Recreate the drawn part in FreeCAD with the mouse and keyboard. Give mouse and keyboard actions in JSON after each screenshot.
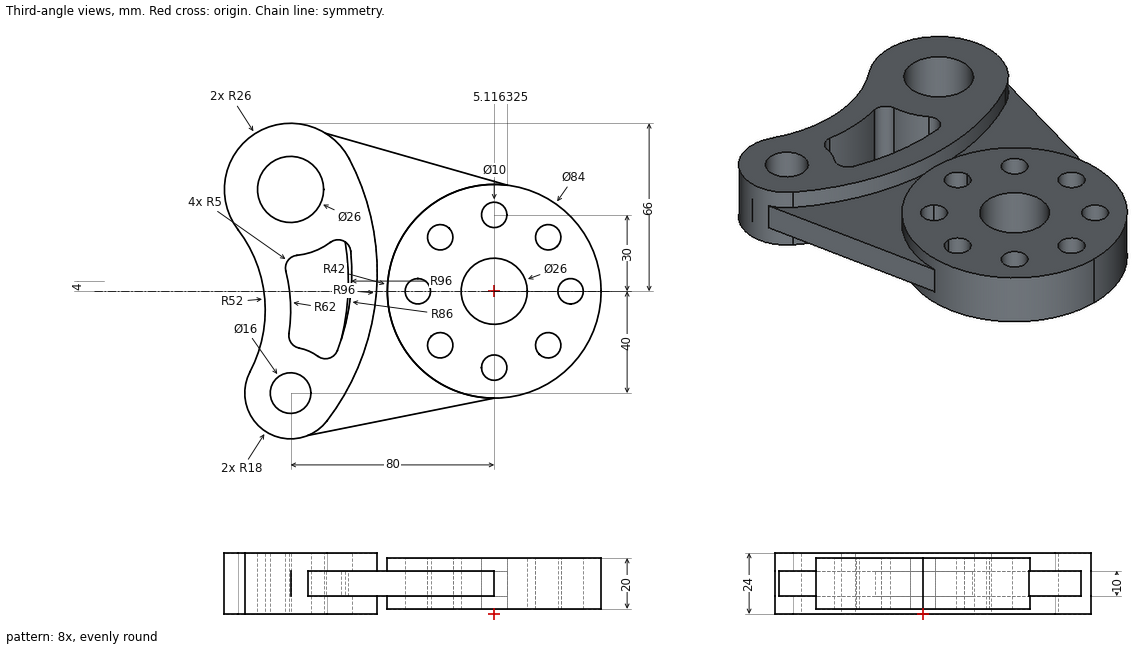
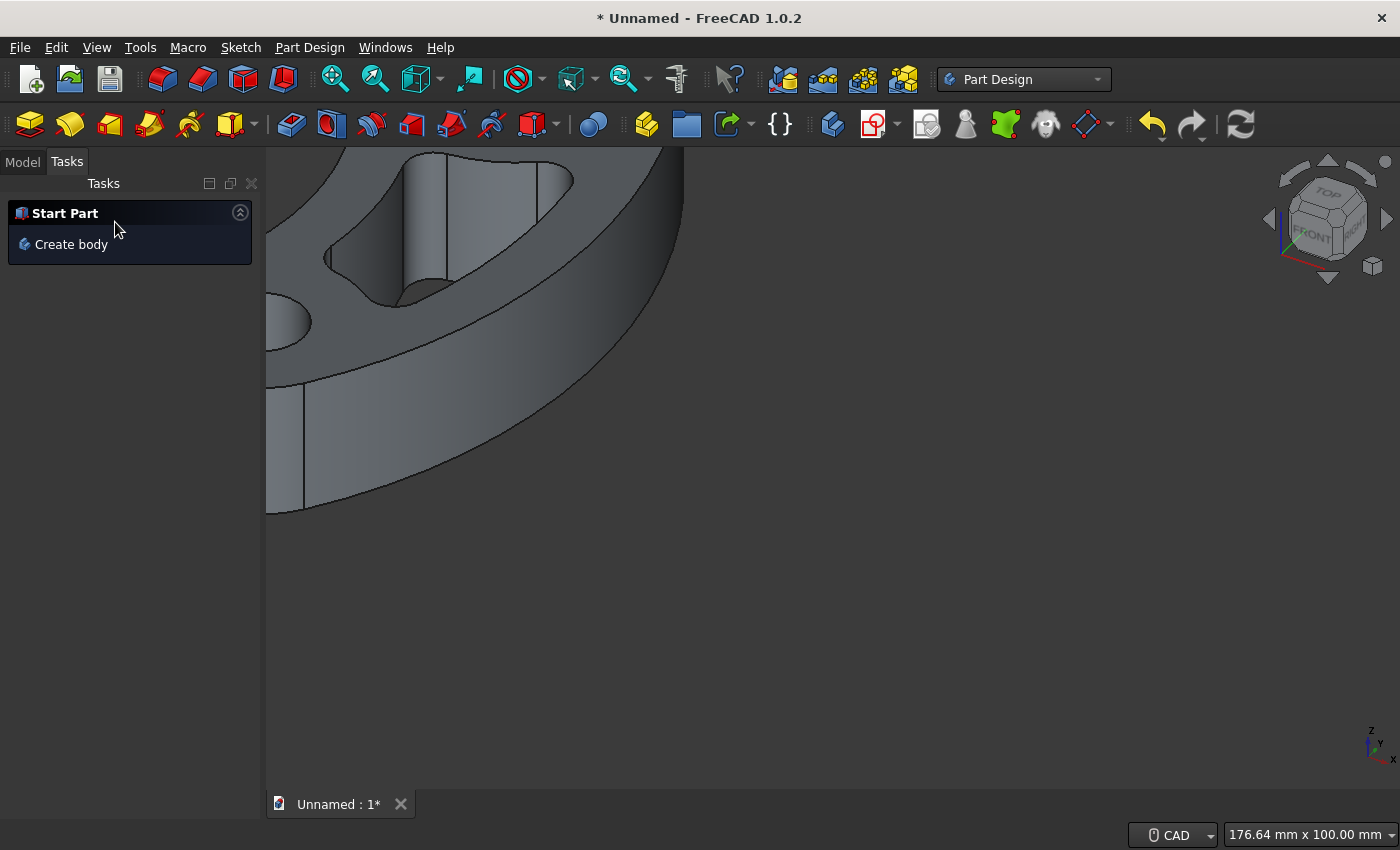
{"action": "left_click", "coordinate": [336, 80]}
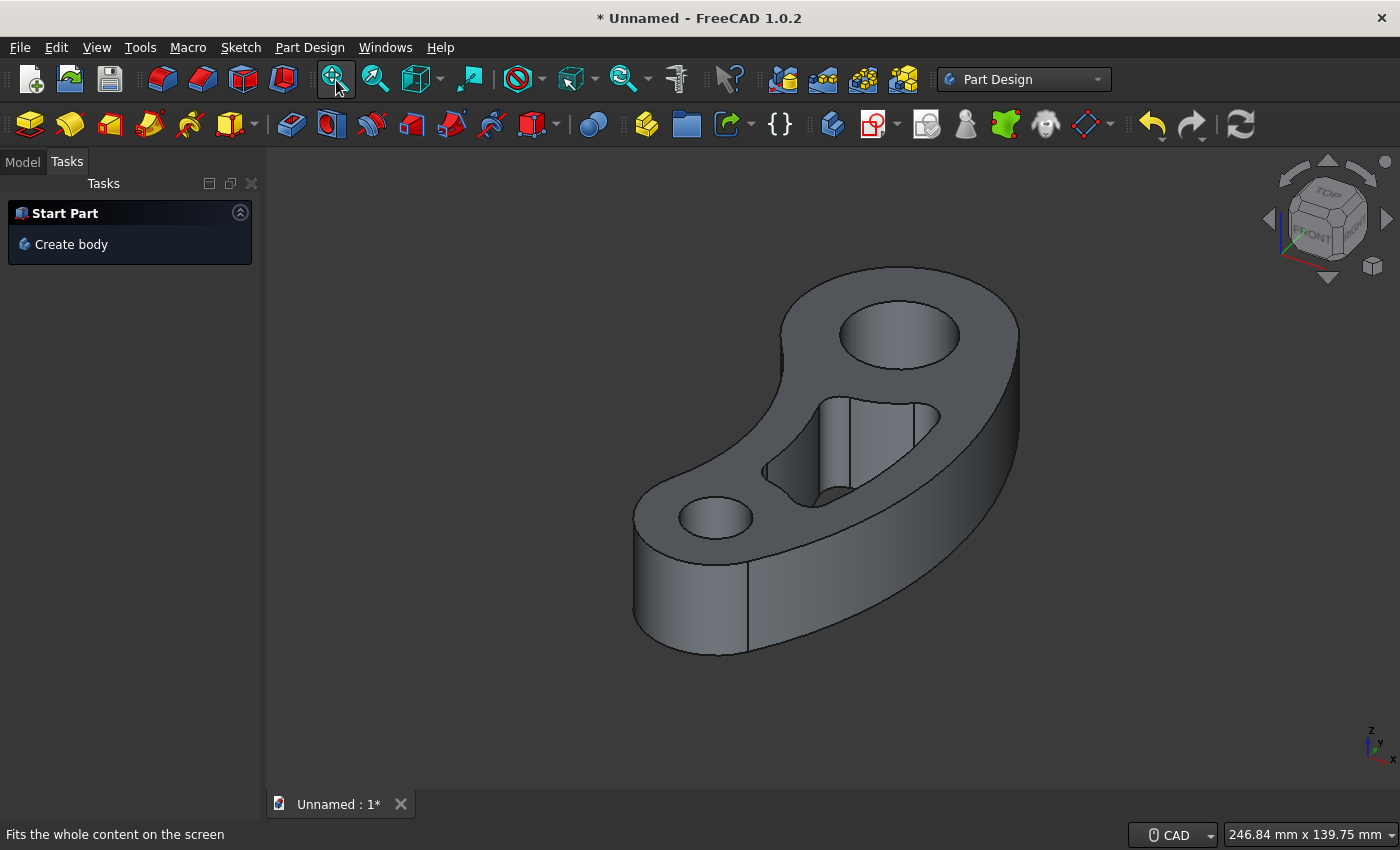
{"action": "left_click", "coordinate": [834, 124]}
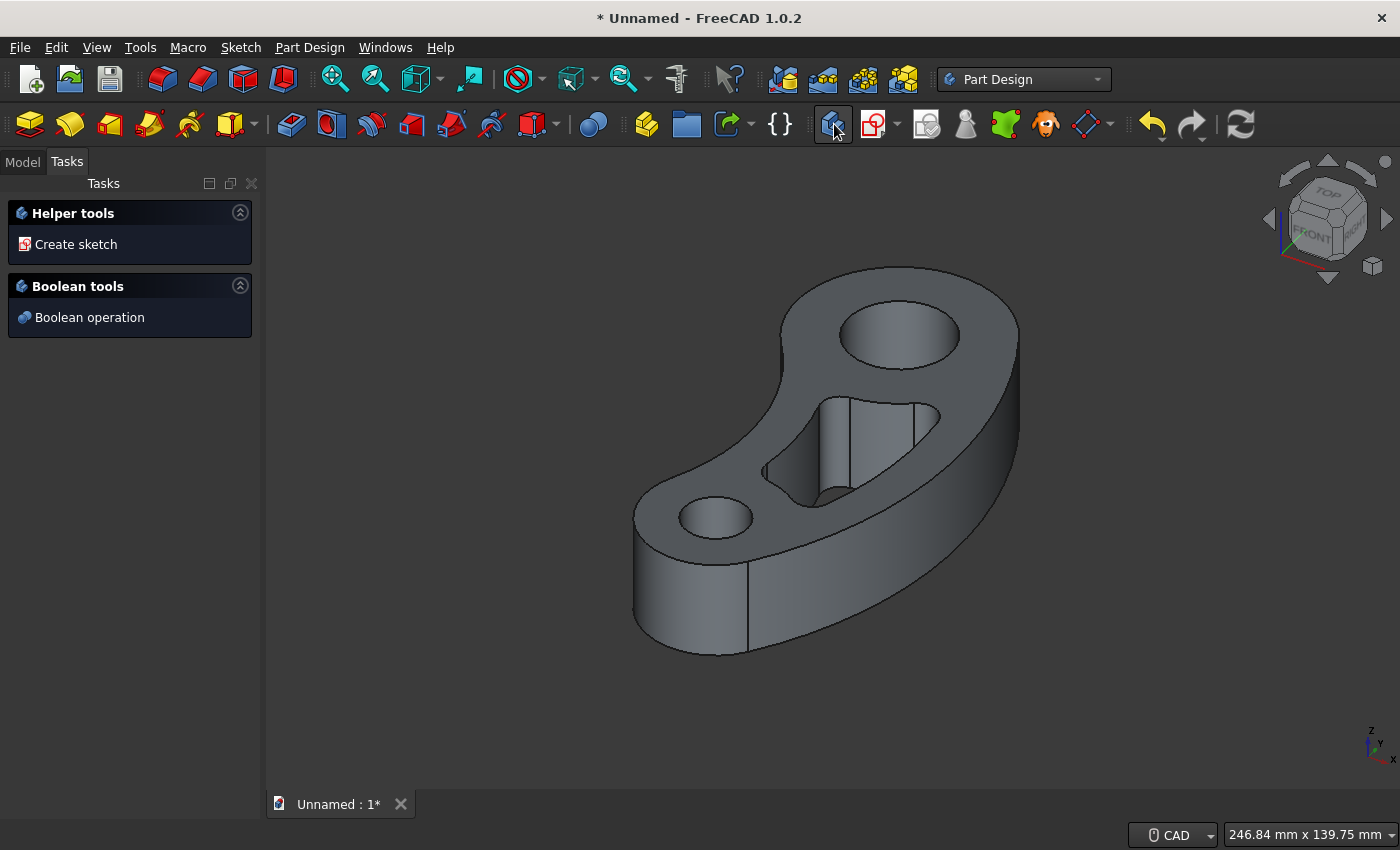
{"action": "left_click", "coordinate": [23, 161]}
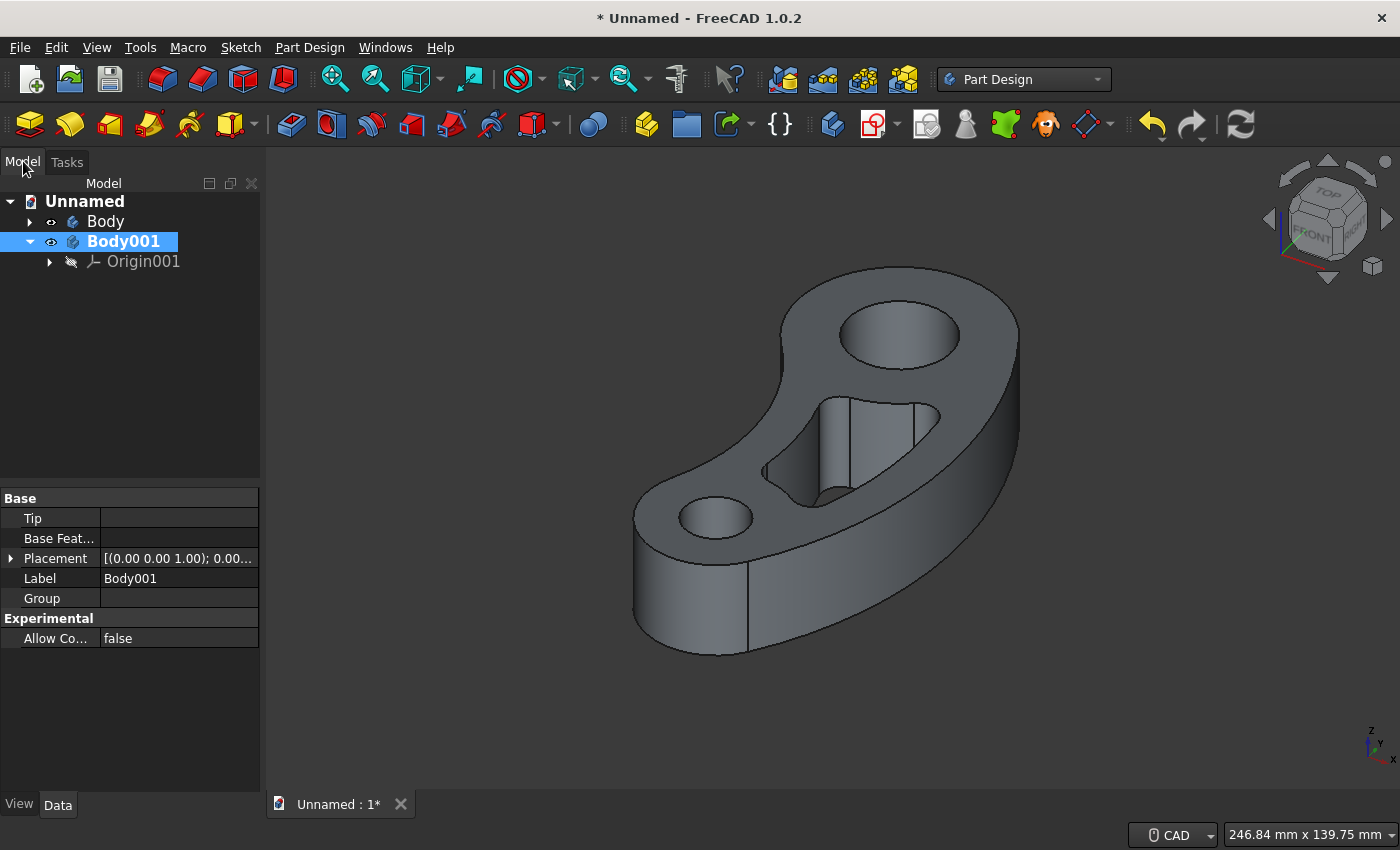
{"action": "left_click", "coordinate": [50, 262]}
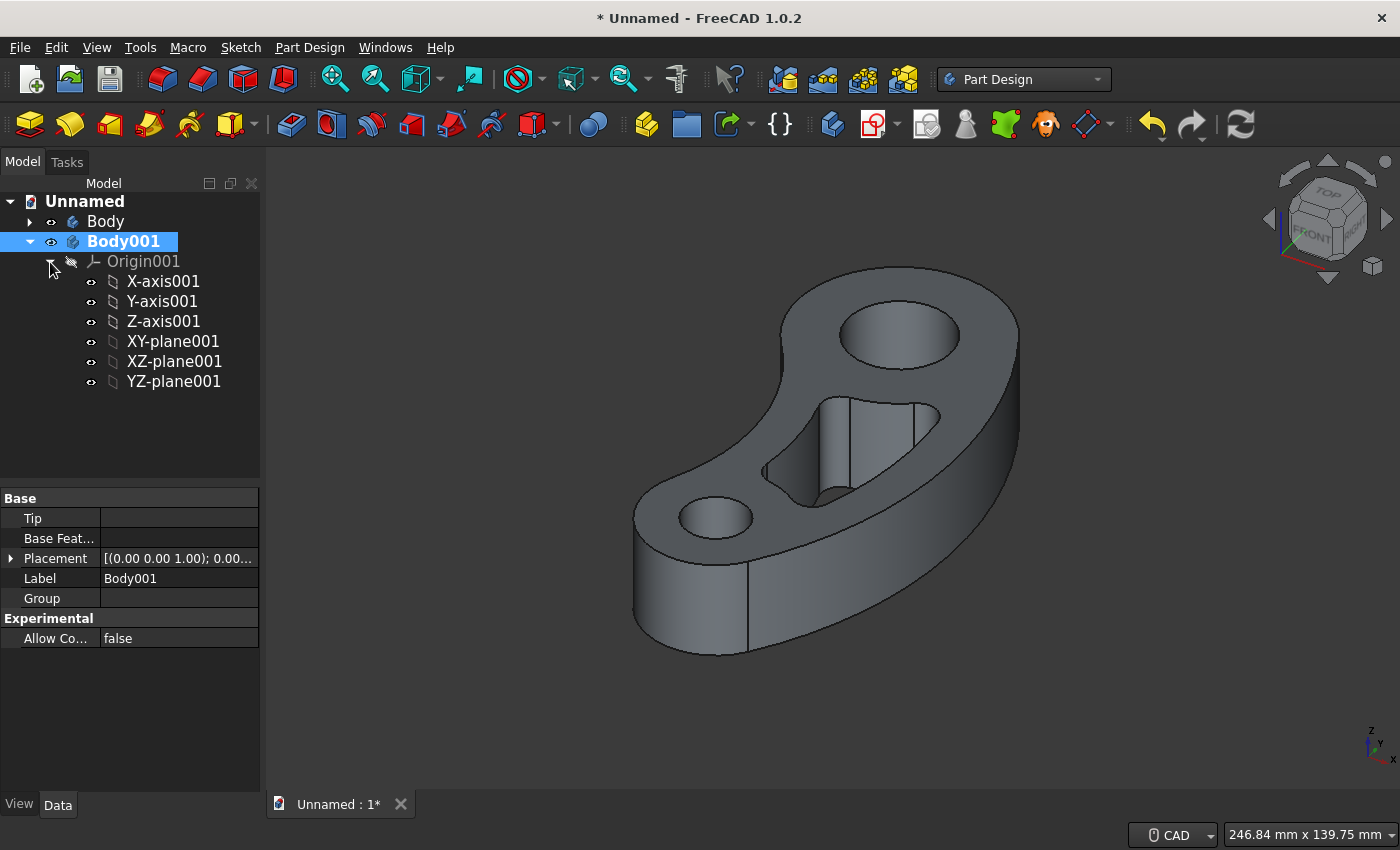
{"action": "left_click", "coordinate": [136, 342]}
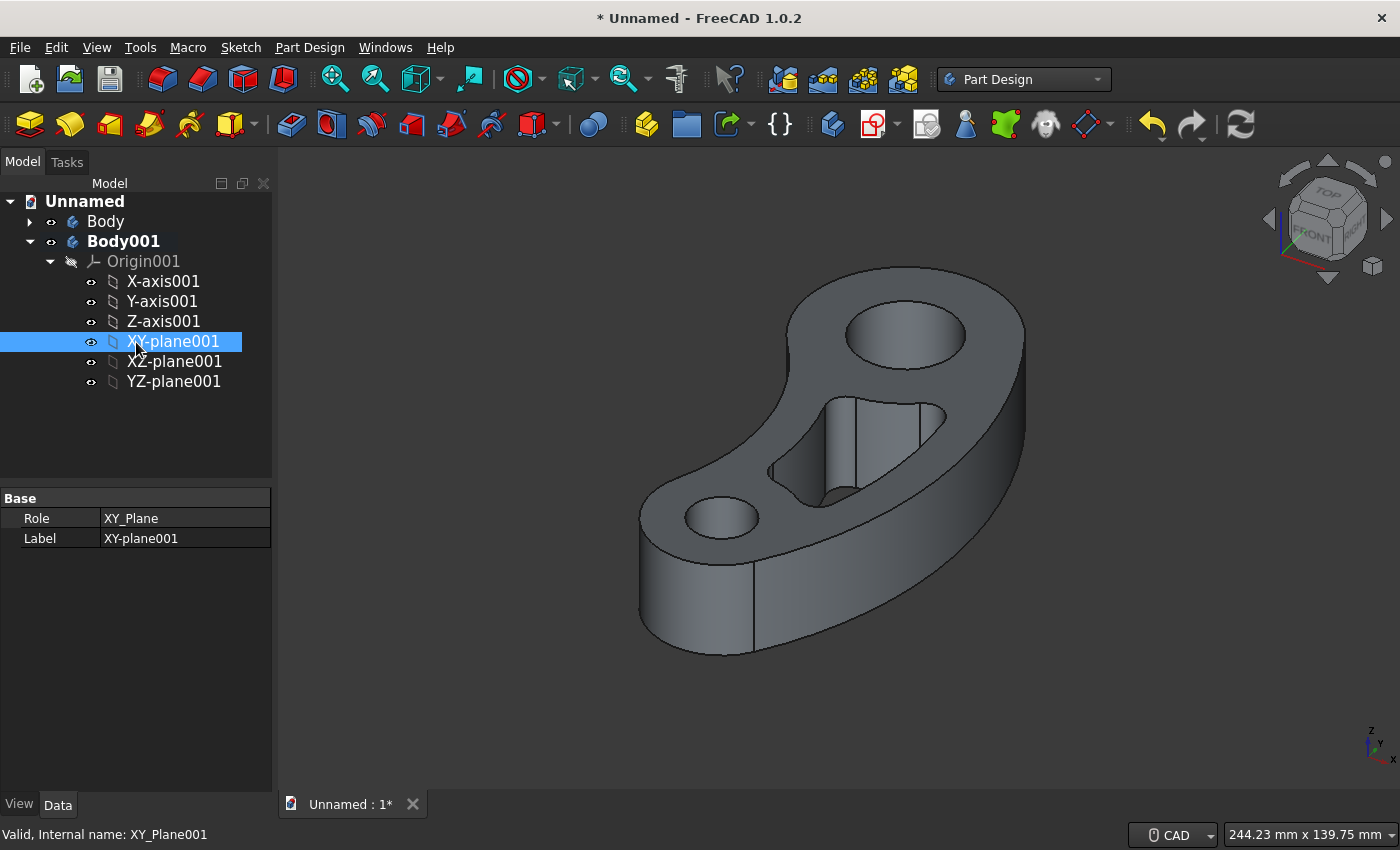
{"action": "left_click", "coordinate": [1086, 124]}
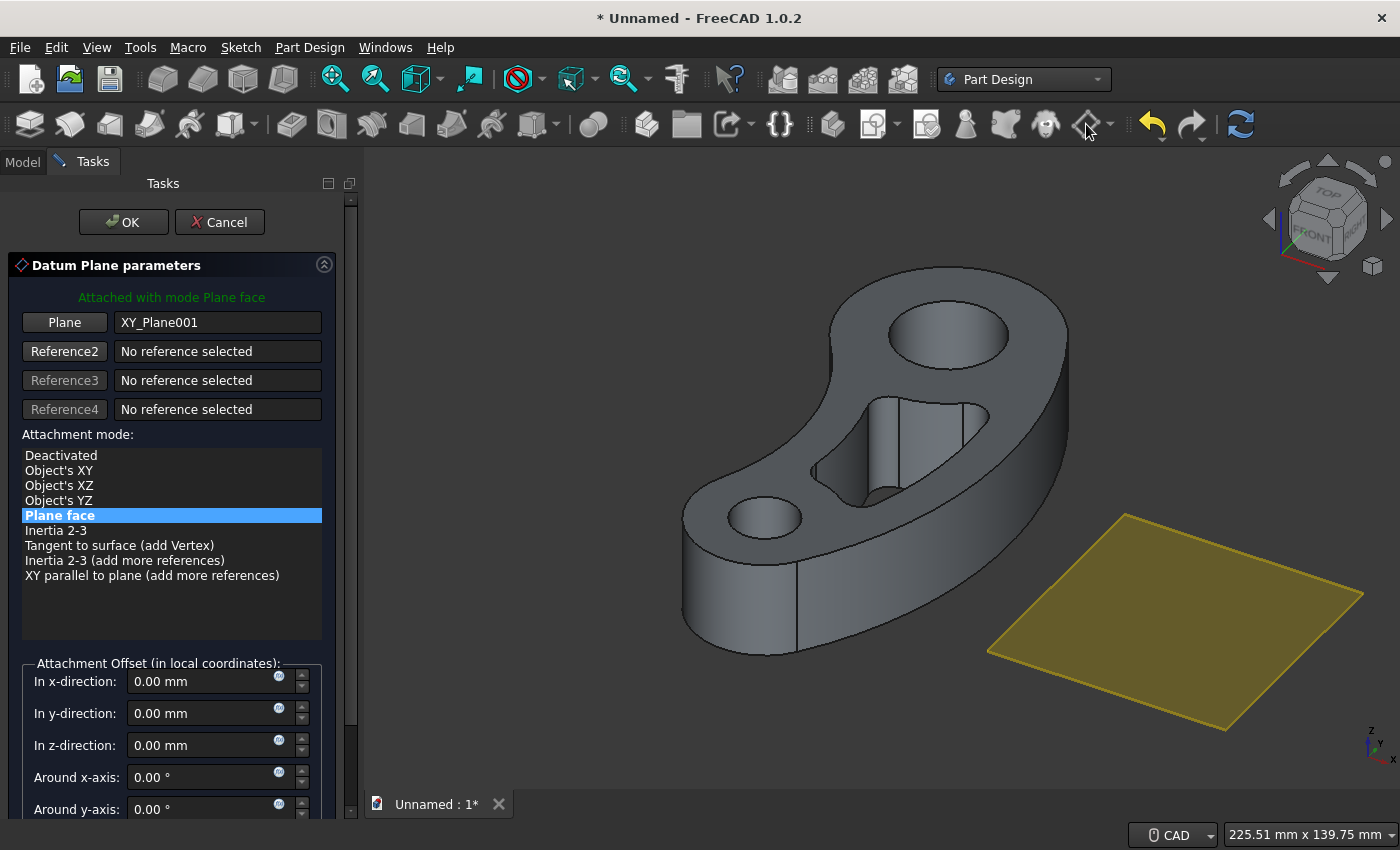
{"action": "triple_click", "coordinate": [210, 745]}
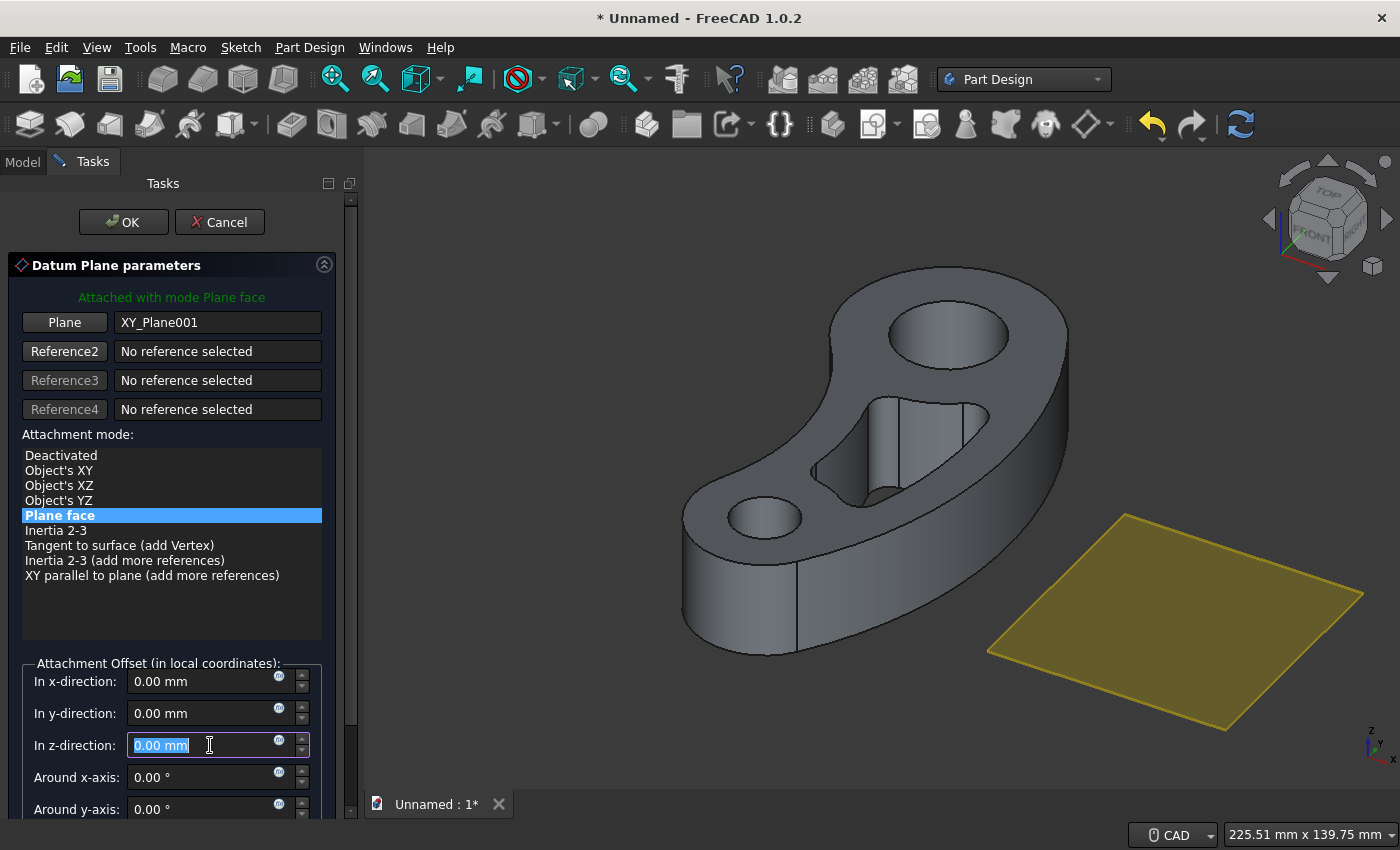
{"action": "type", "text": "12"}
{"action": "key", "text": "Tab"}